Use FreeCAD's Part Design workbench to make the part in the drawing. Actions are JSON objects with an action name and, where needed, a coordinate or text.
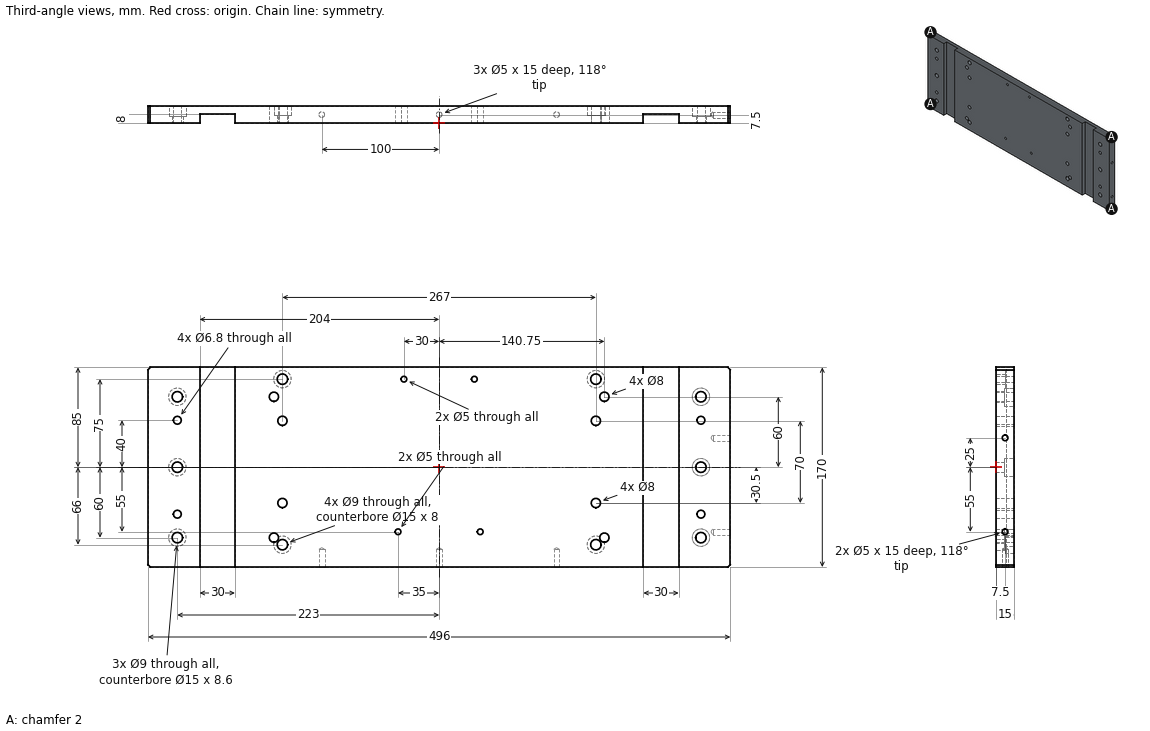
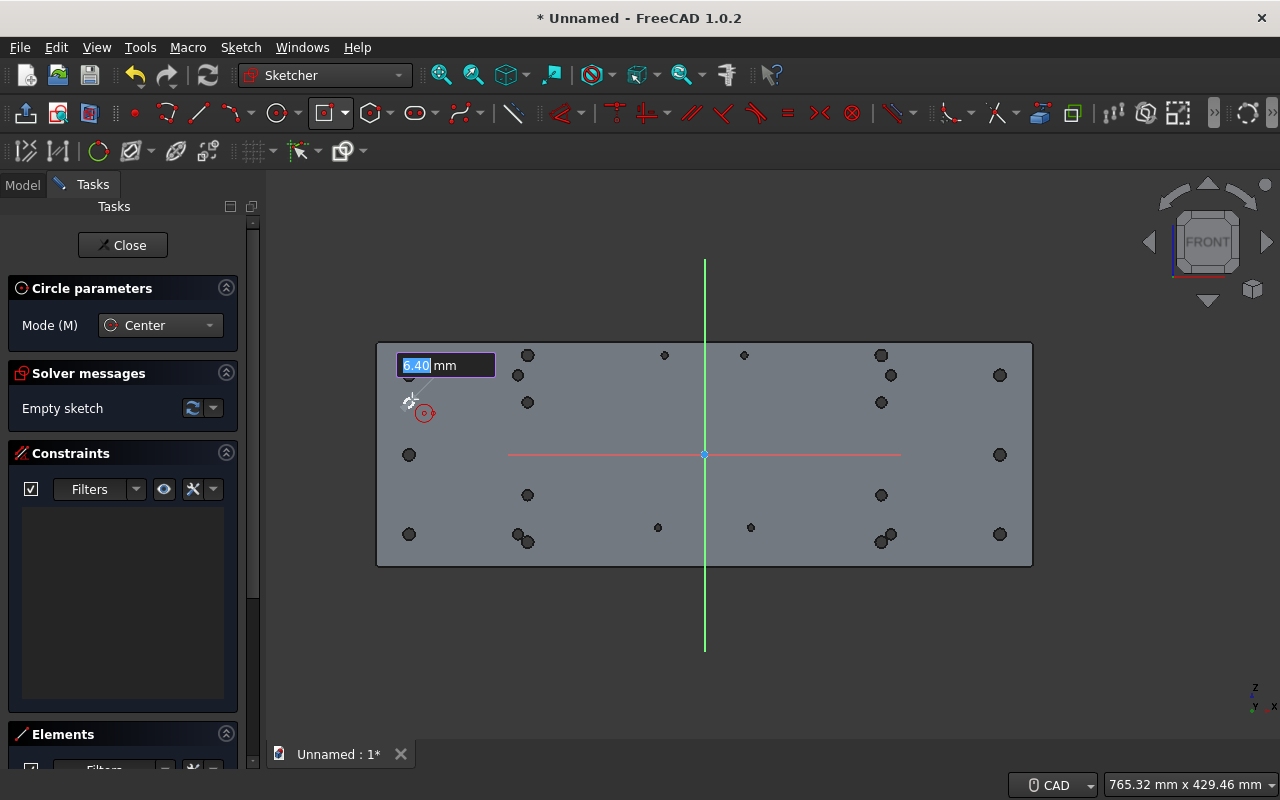
{"action": "type", "text": "6.8"}
{"action": "key", "text": "Return"}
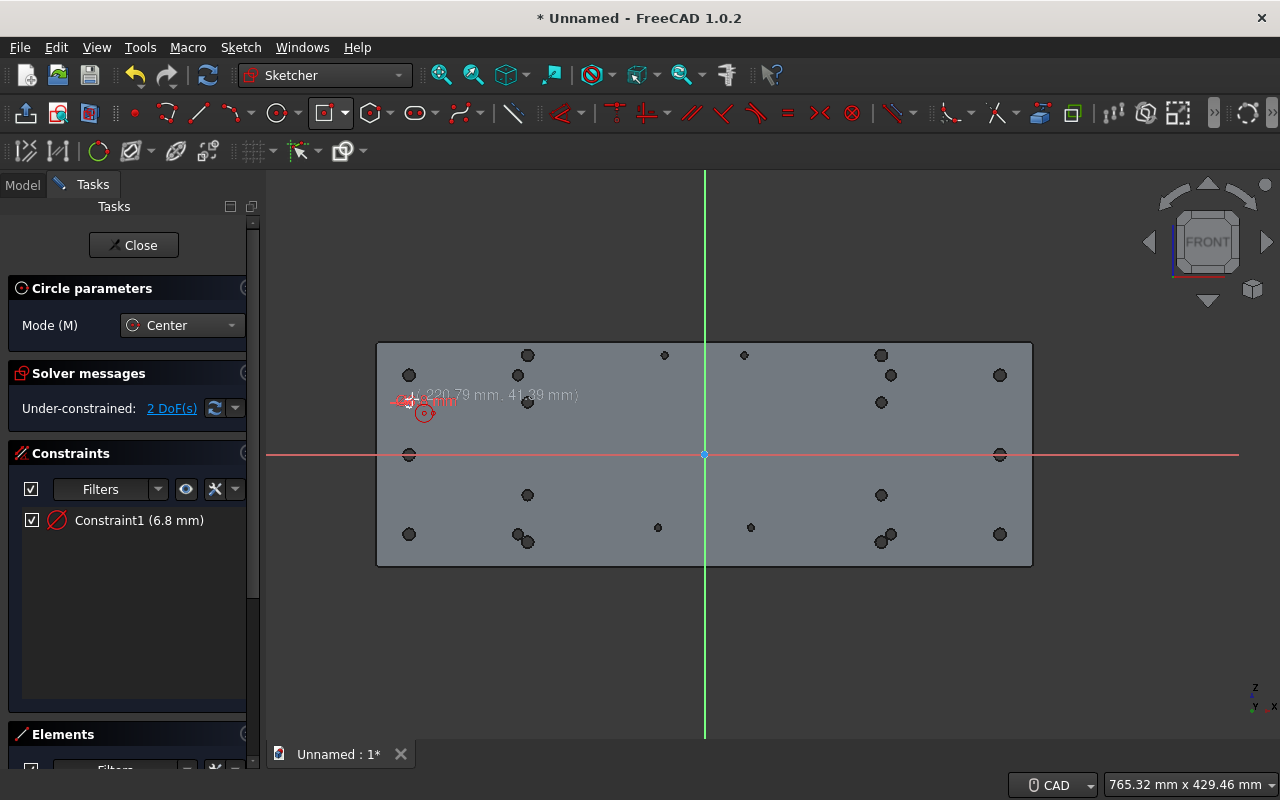
{"action": "scroll", "coordinate": [409, 508], "scroll_direction": "up", "scroll_amount": 9}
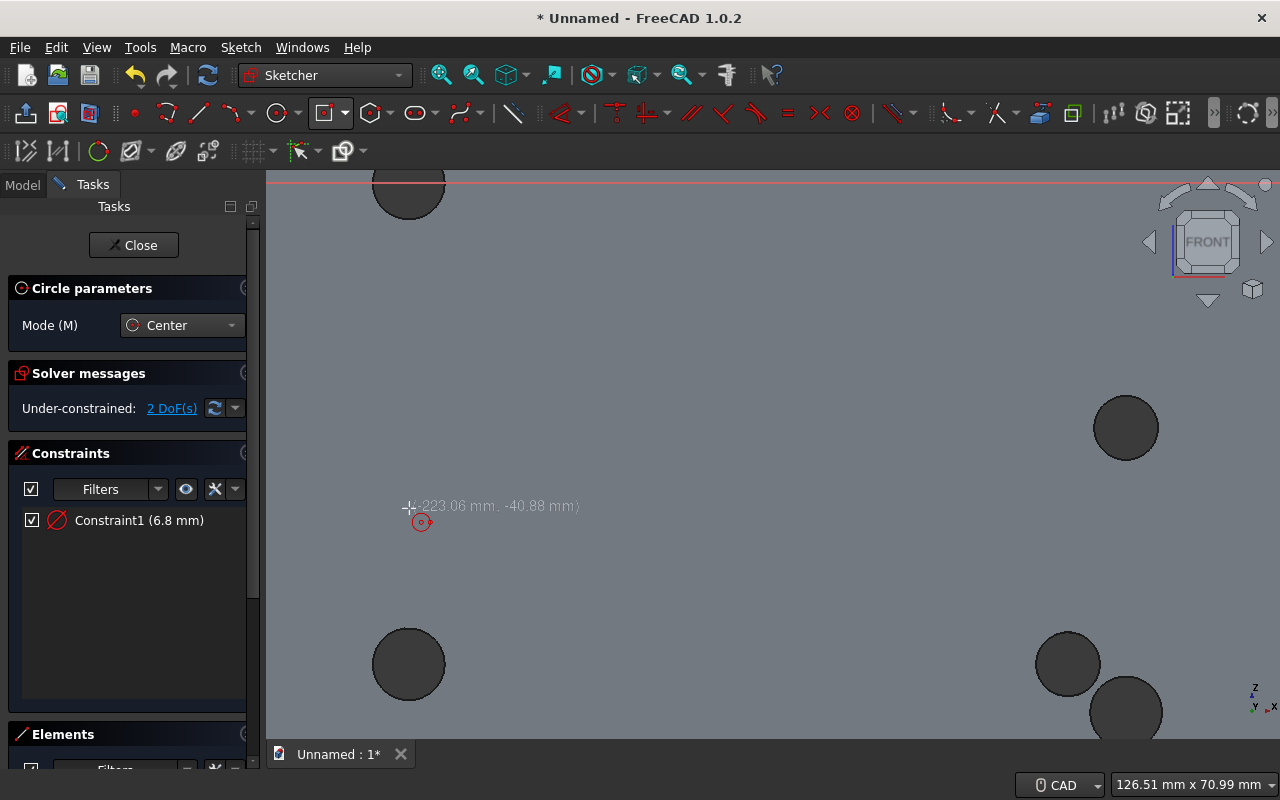
{"action": "scroll", "coordinate": [409, 508], "scroll_direction": "down", "scroll_amount": 9}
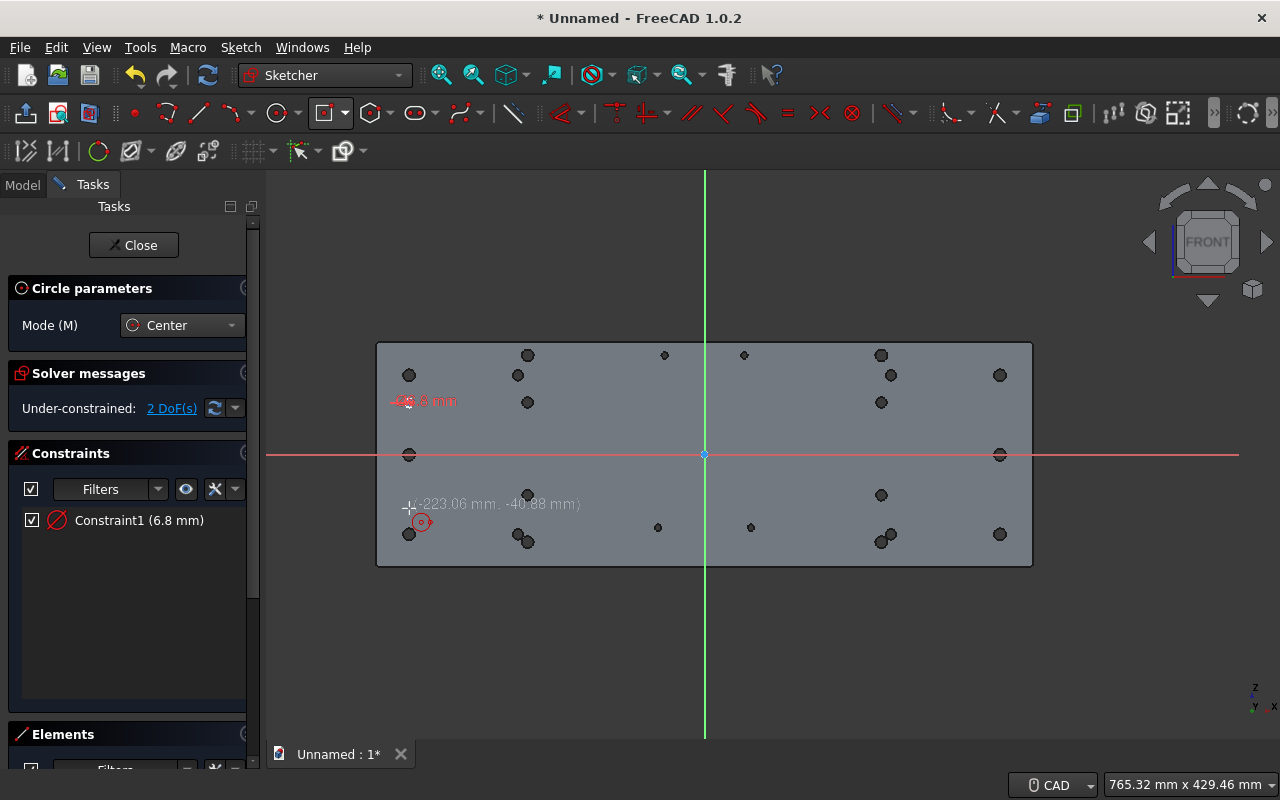
{"action": "left_click", "coordinate": [409, 508]}
{"action": "mouse_move", "coordinate": [412, 505]}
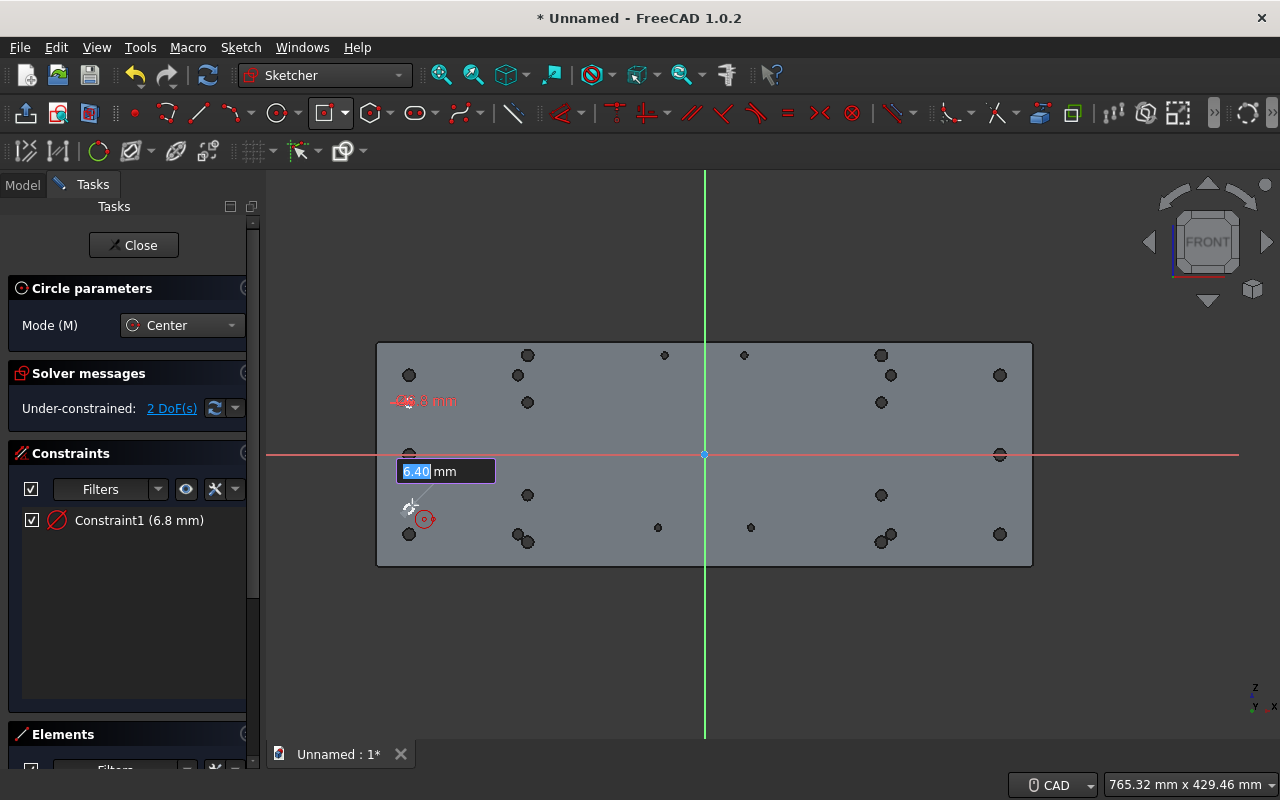
{"action": "type", "text": "6.8"}
{"action": "key", "text": "Return"}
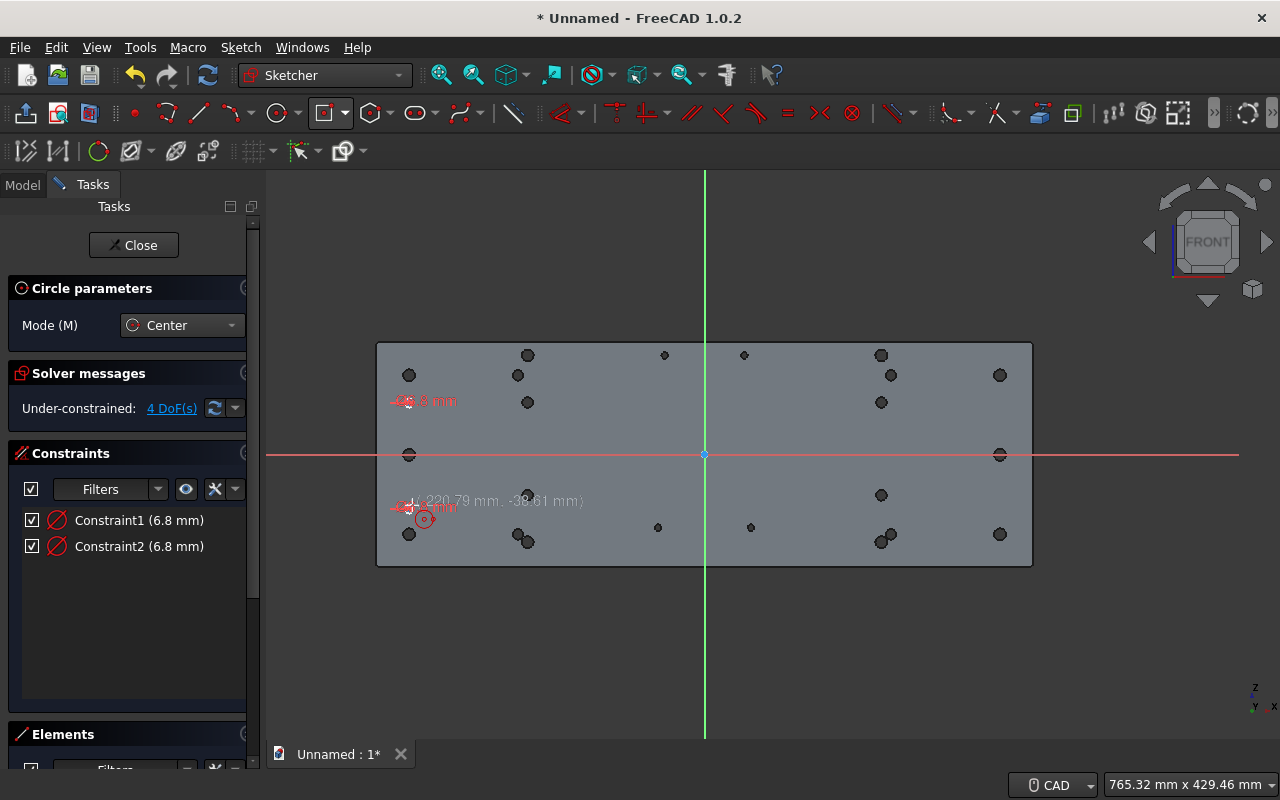
{"action": "scroll", "coordinate": [1000, 508], "scroll_direction": "up", "scroll_amount": 9}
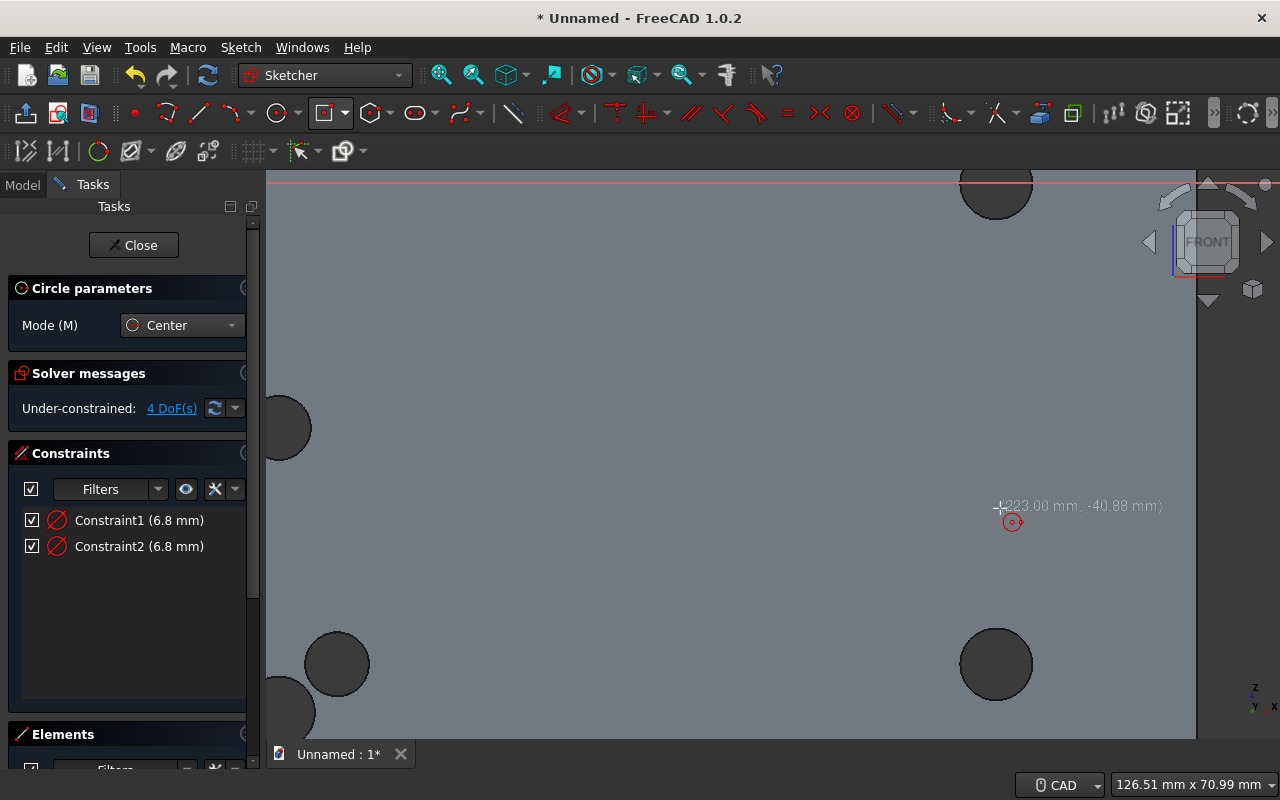
{"action": "scroll", "coordinate": [1001, 508], "scroll_direction": "down", "scroll_amount": 9}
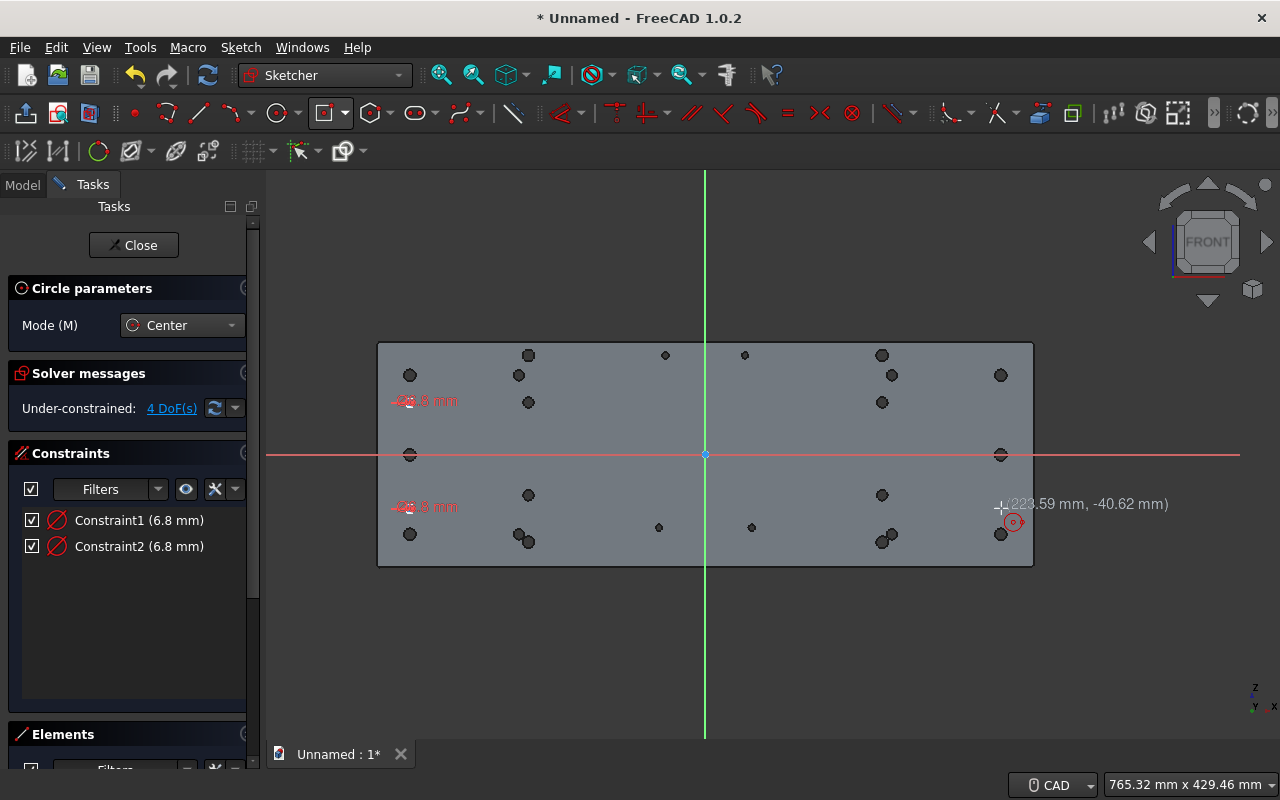
{"action": "left_click", "coordinate": [1001, 508]}
{"action": "mouse_move", "coordinate": [1004, 505]}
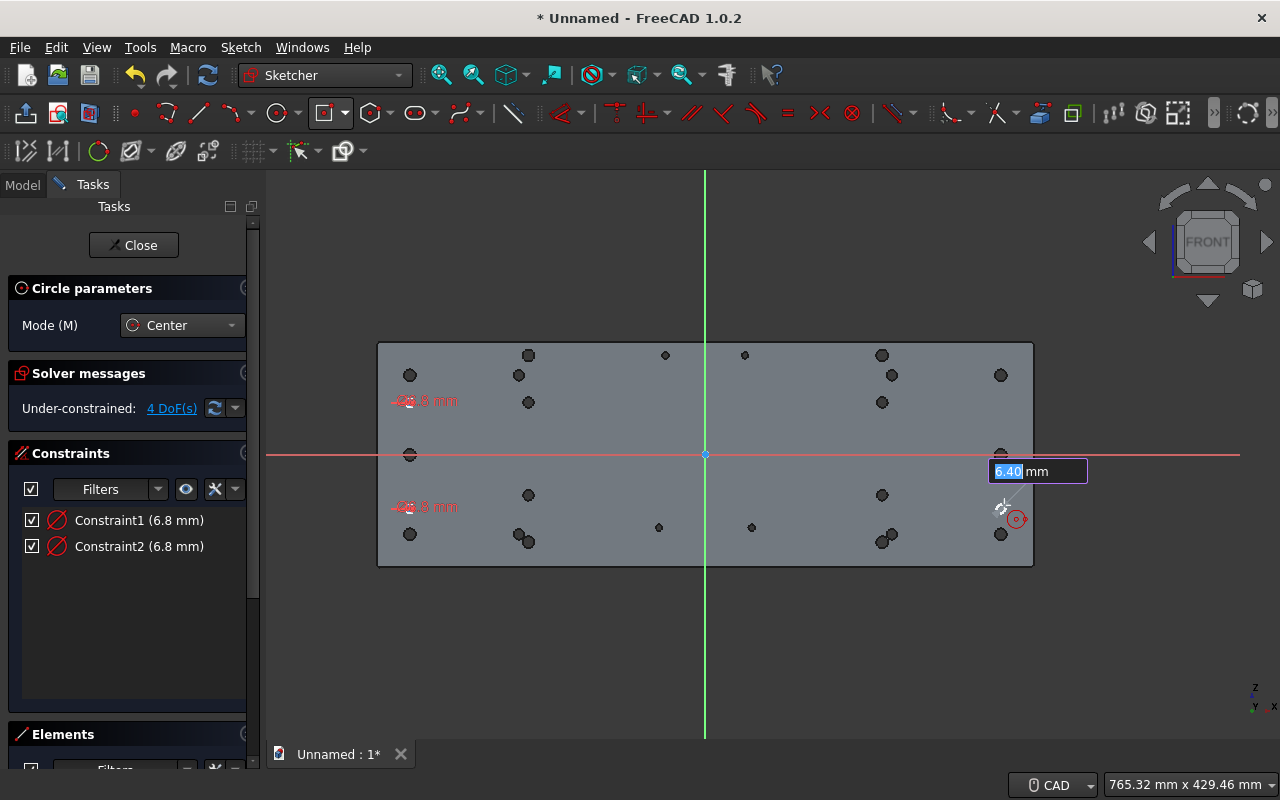
{"action": "type", "text": "6.8"}
{"action": "key", "text": "Return"}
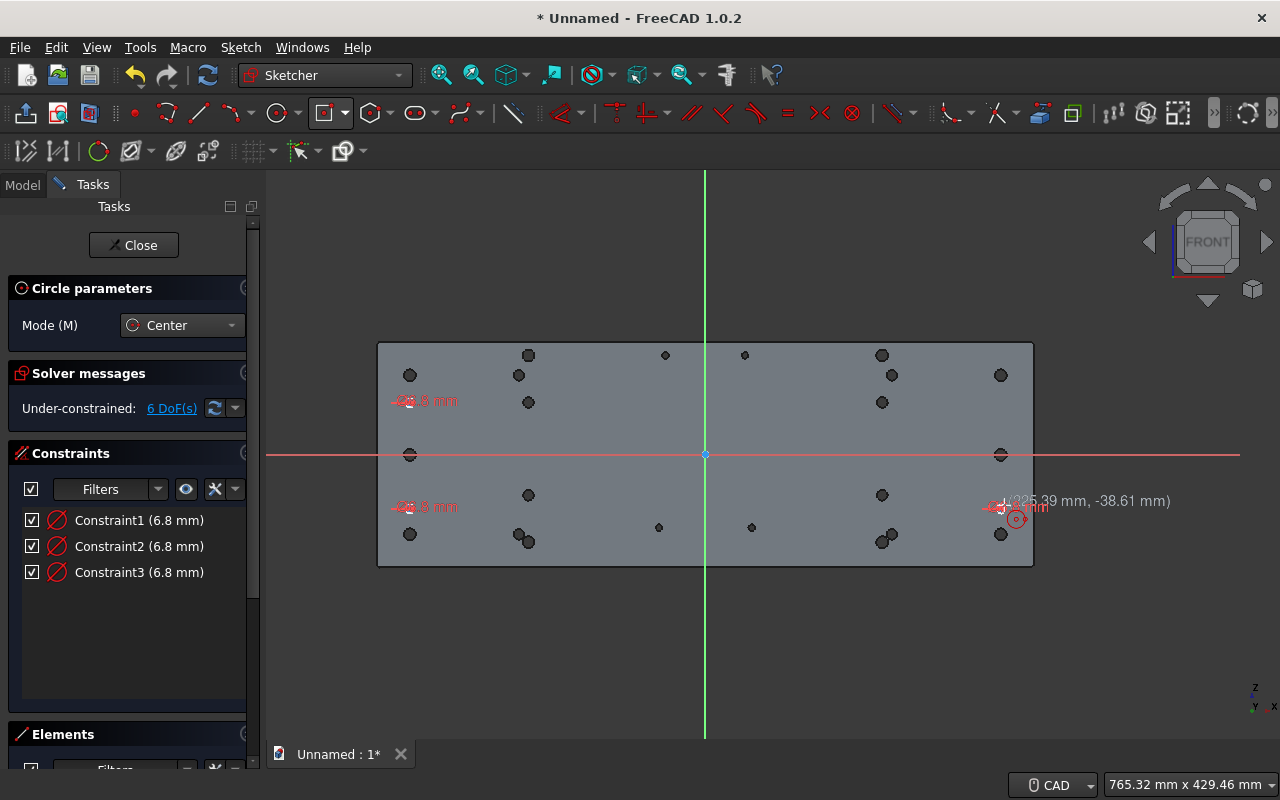
{"action": "scroll", "coordinate": [1001, 402], "scroll_direction": "up", "scroll_amount": 9}